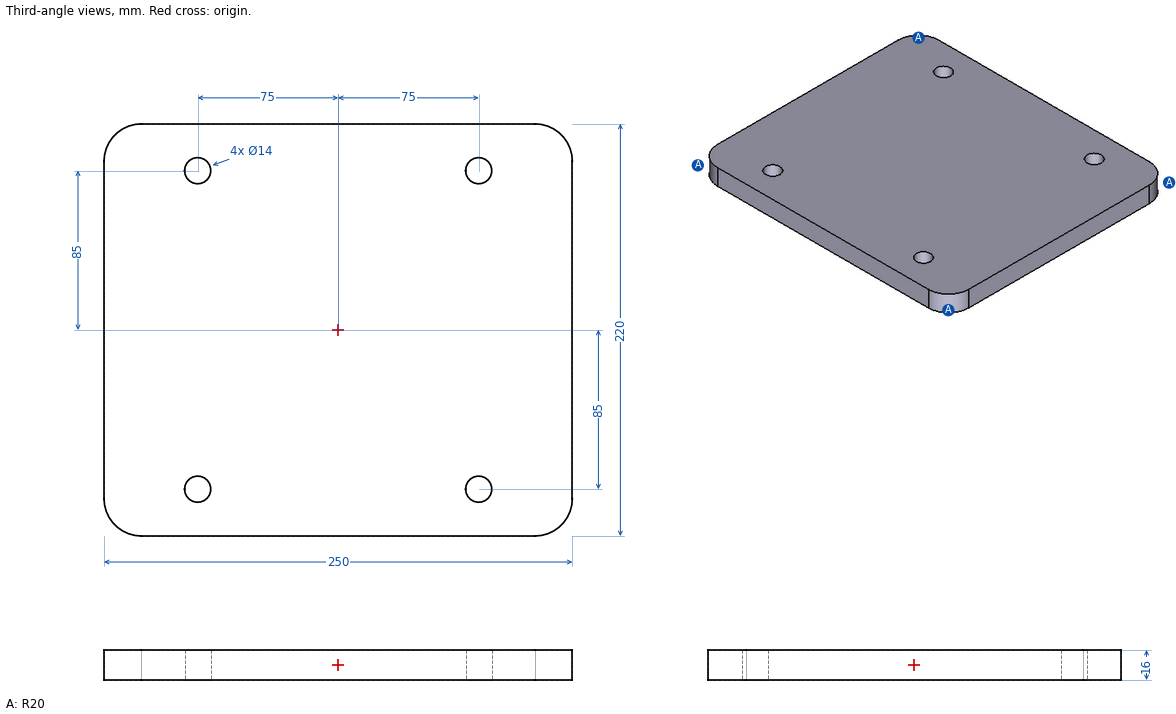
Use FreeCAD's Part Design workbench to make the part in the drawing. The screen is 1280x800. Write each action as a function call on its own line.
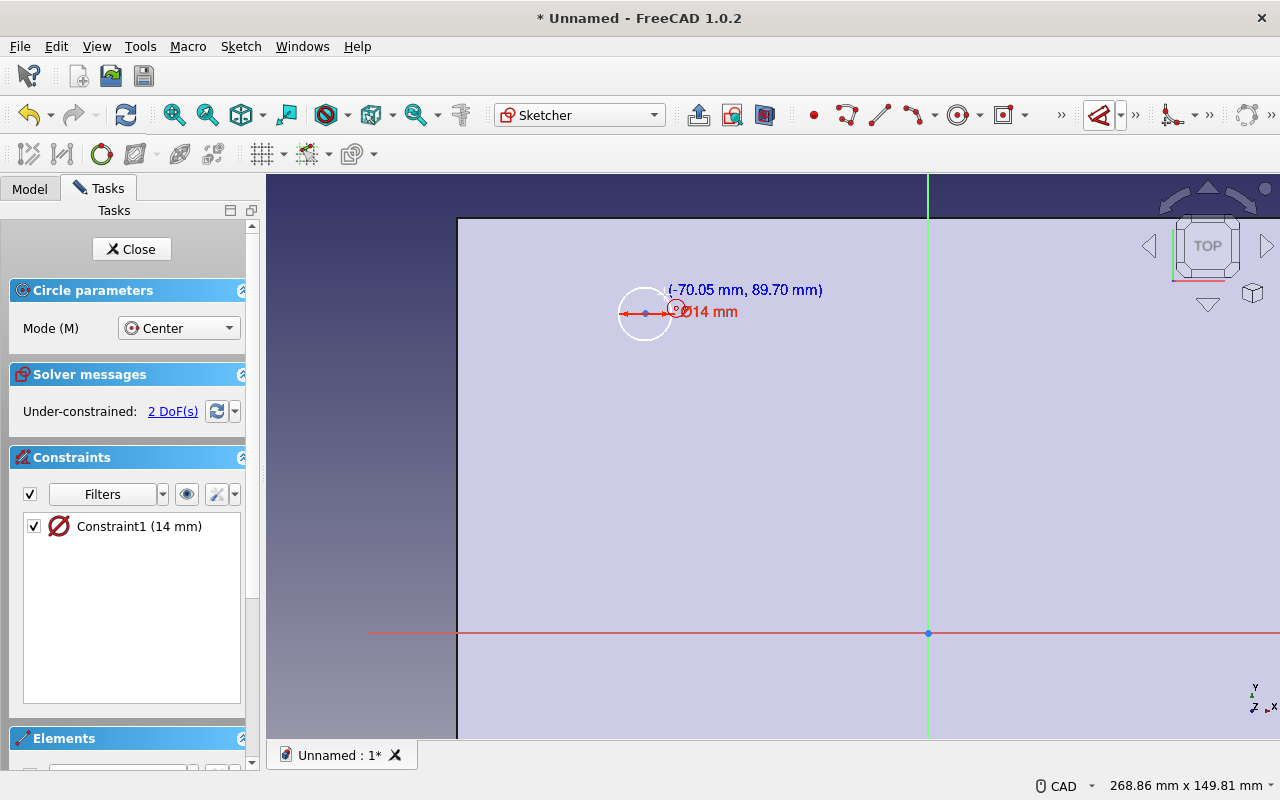
scroll(432, 241, down, 3)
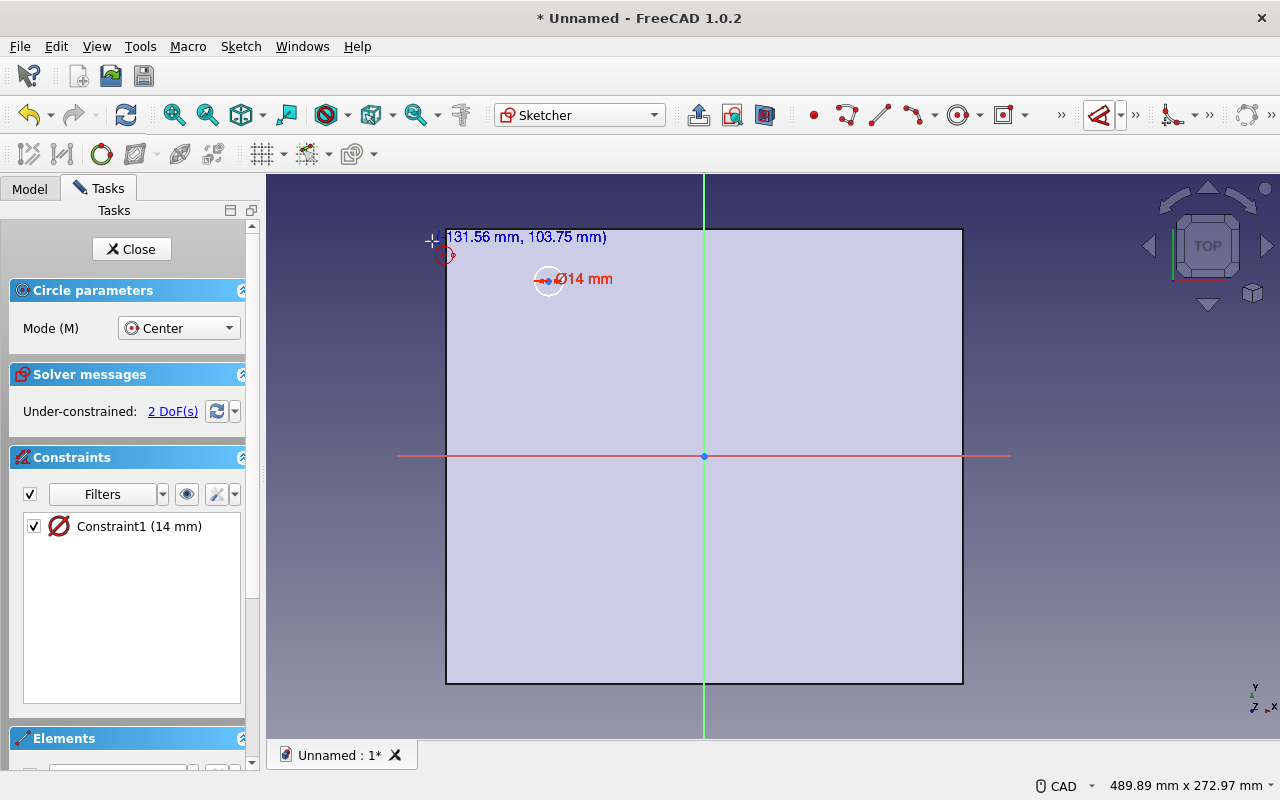
scroll(860, 280, up, 3)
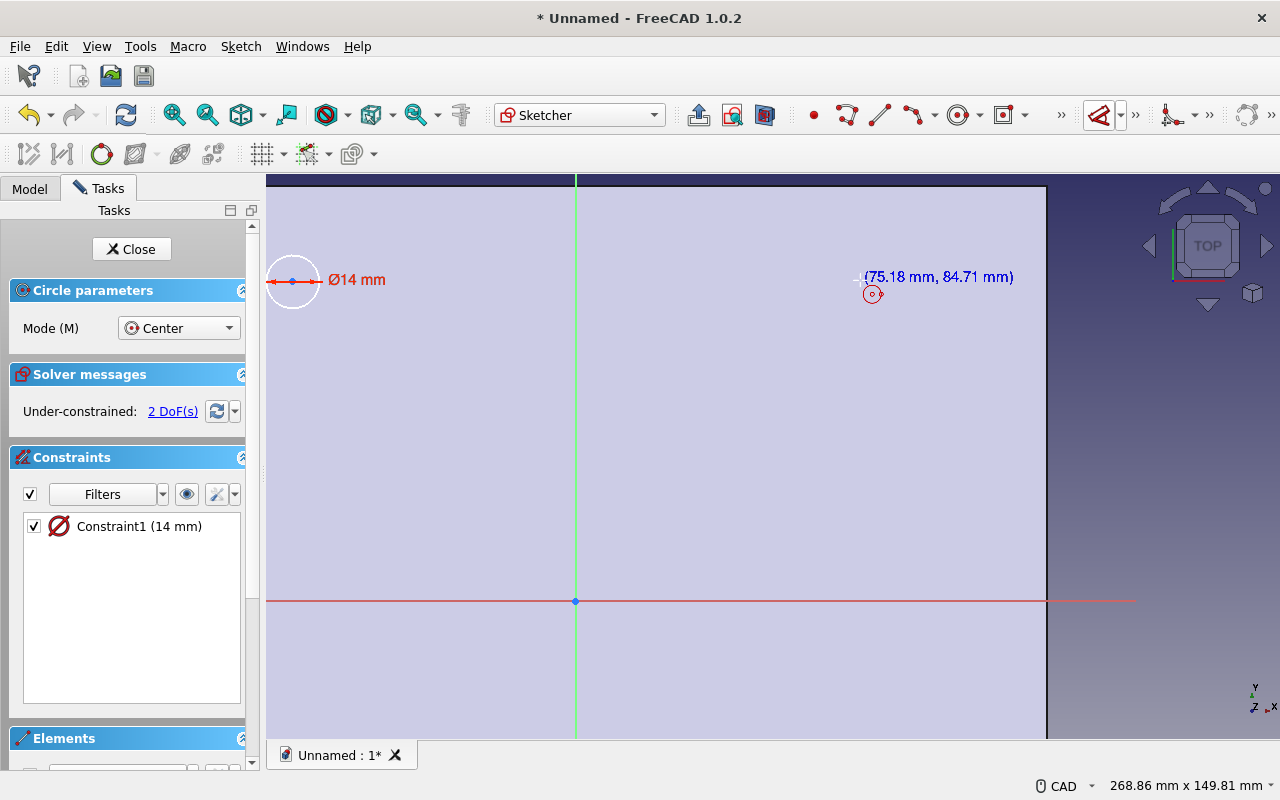
click(859, 281)
move(878, 262)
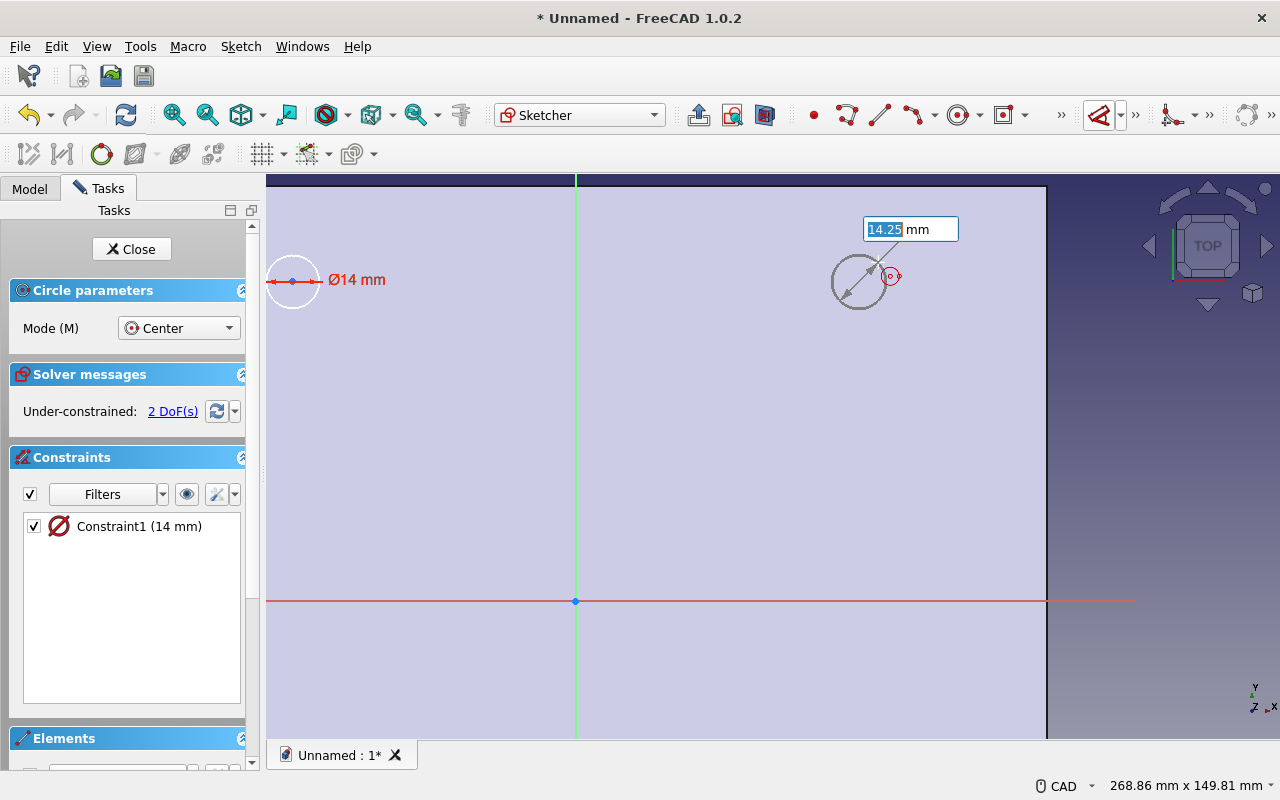
text(14)
key(Return)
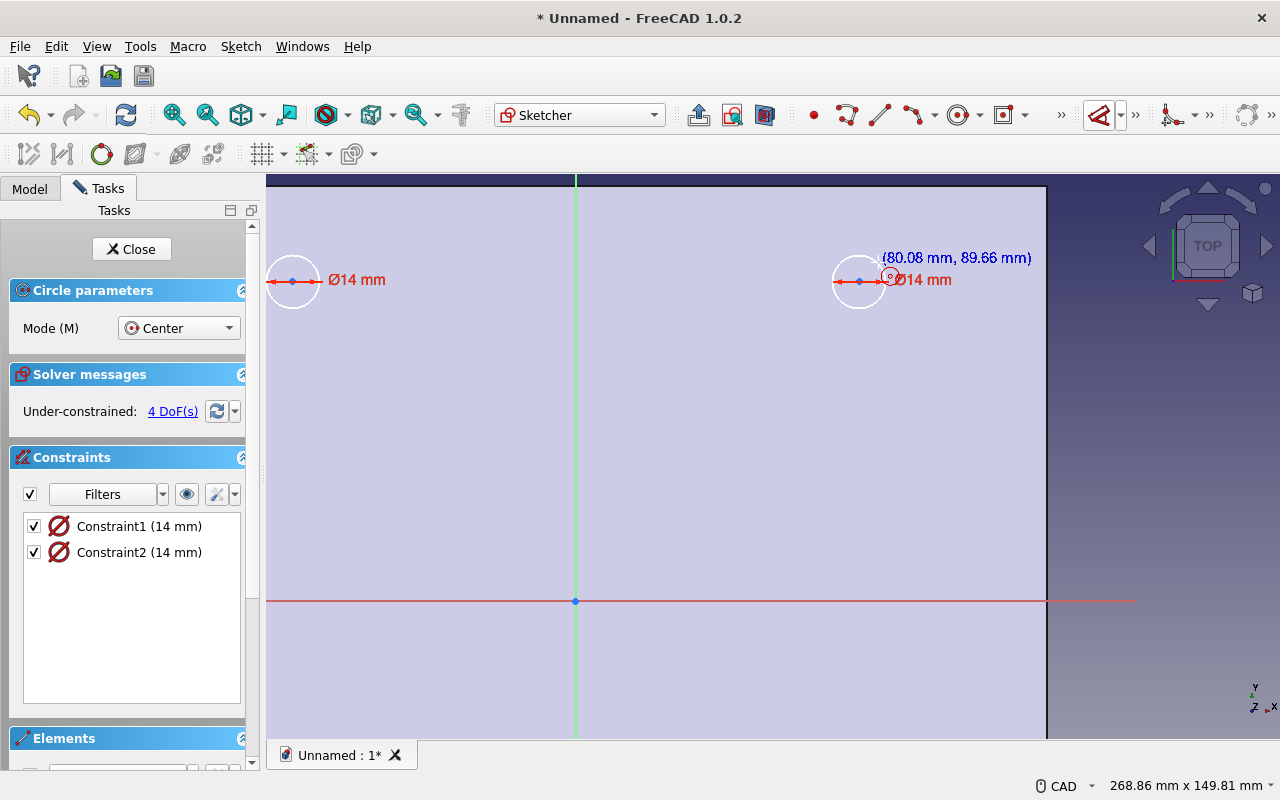
scroll(861, 281, down, 3)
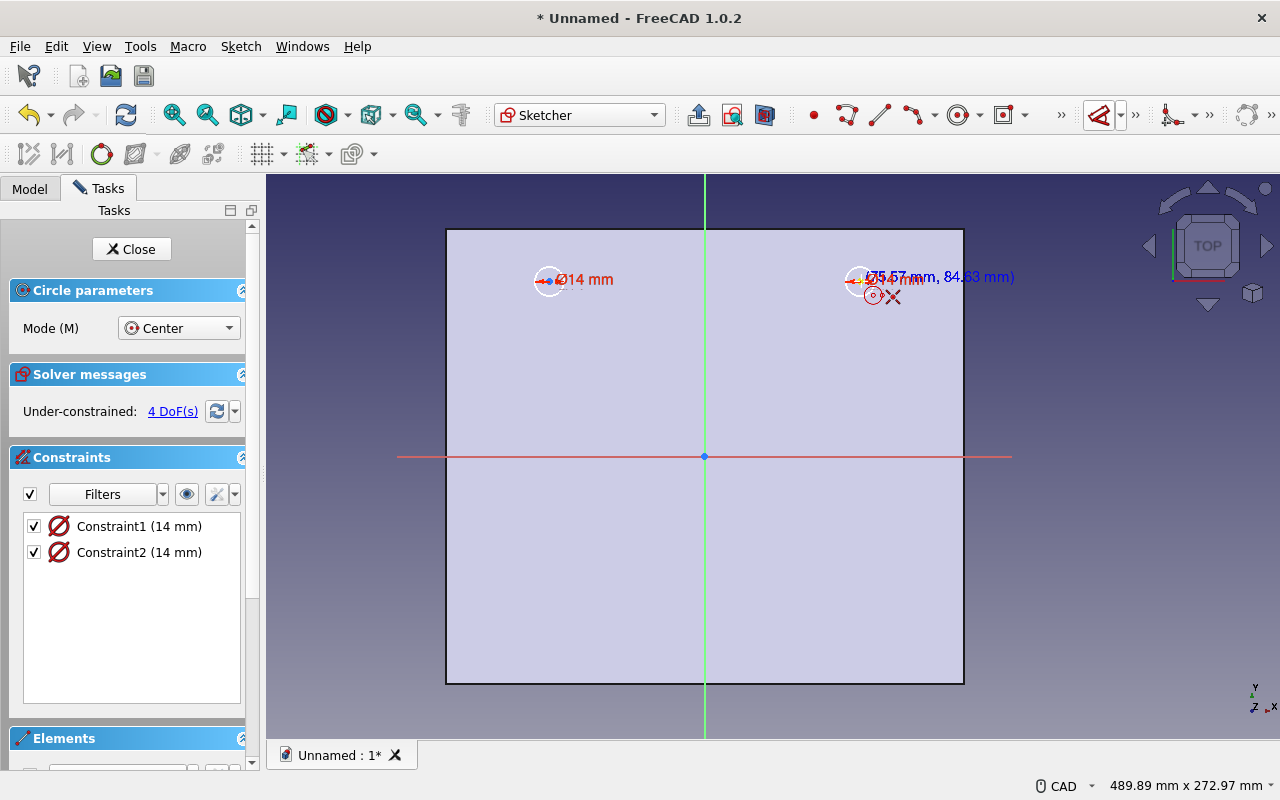
scroll(860, 633, up, 3)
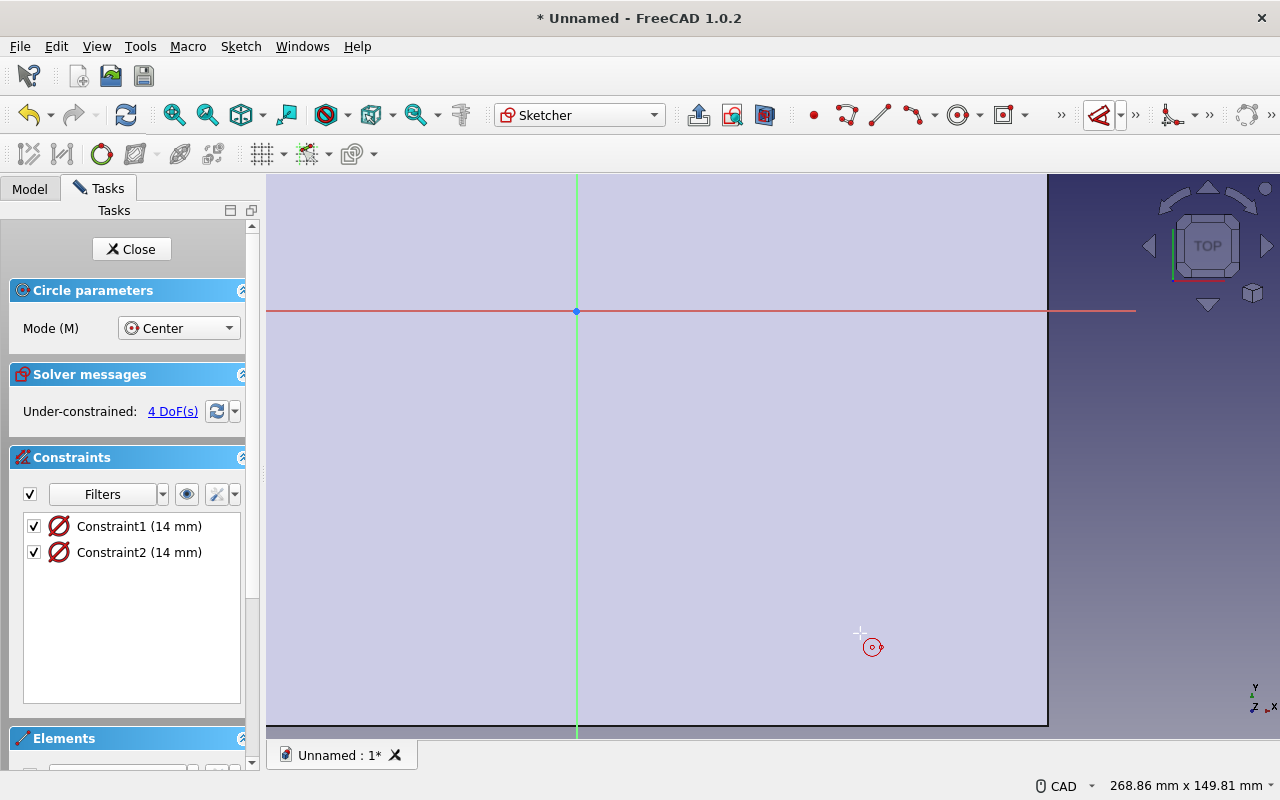
click(860, 632)
move(878, 613)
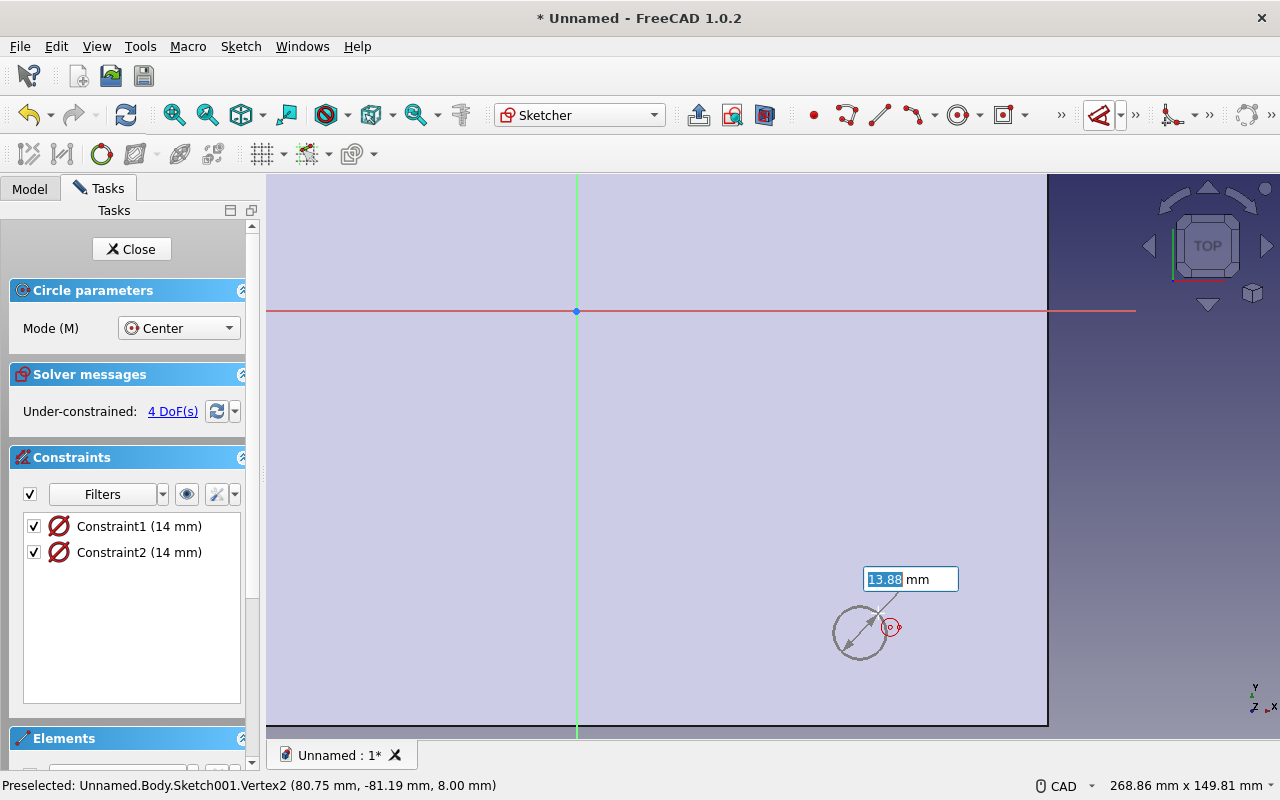
text(14)
key(Return)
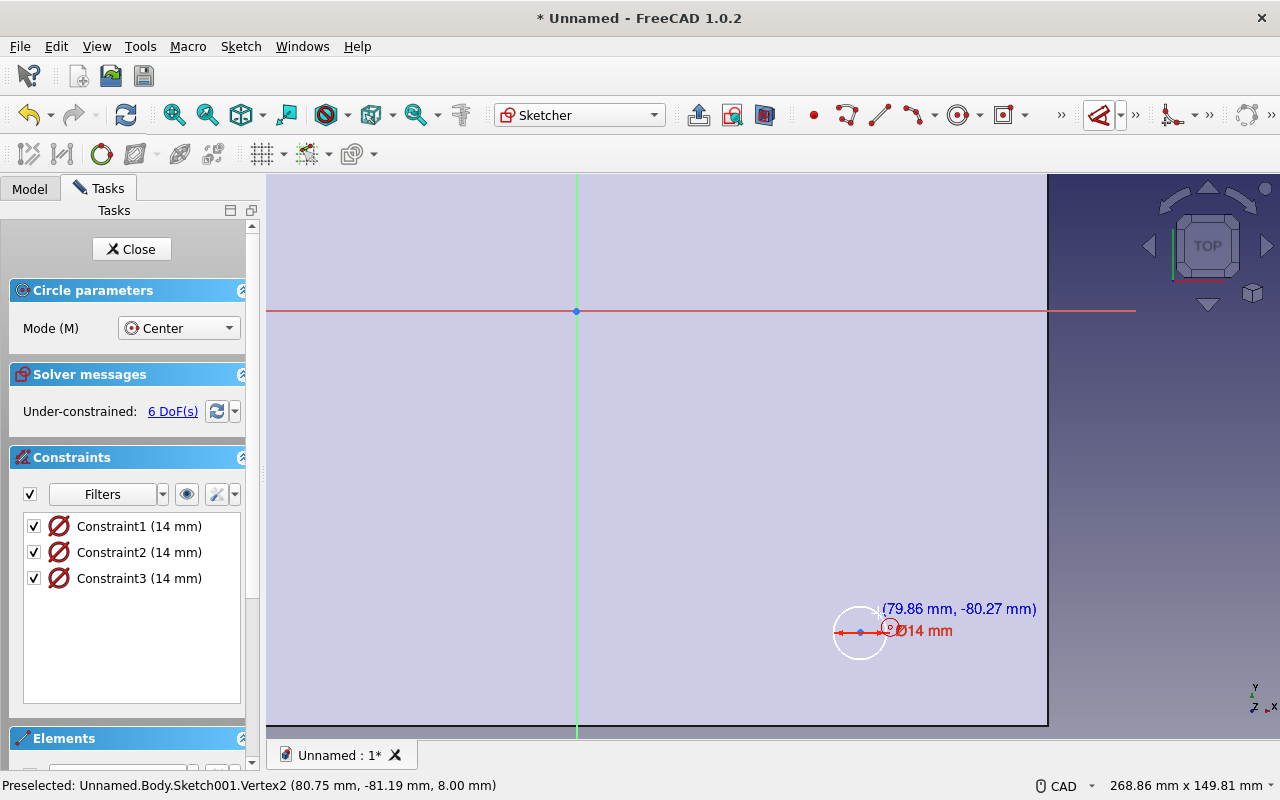
scroll(860, 633, down, 3)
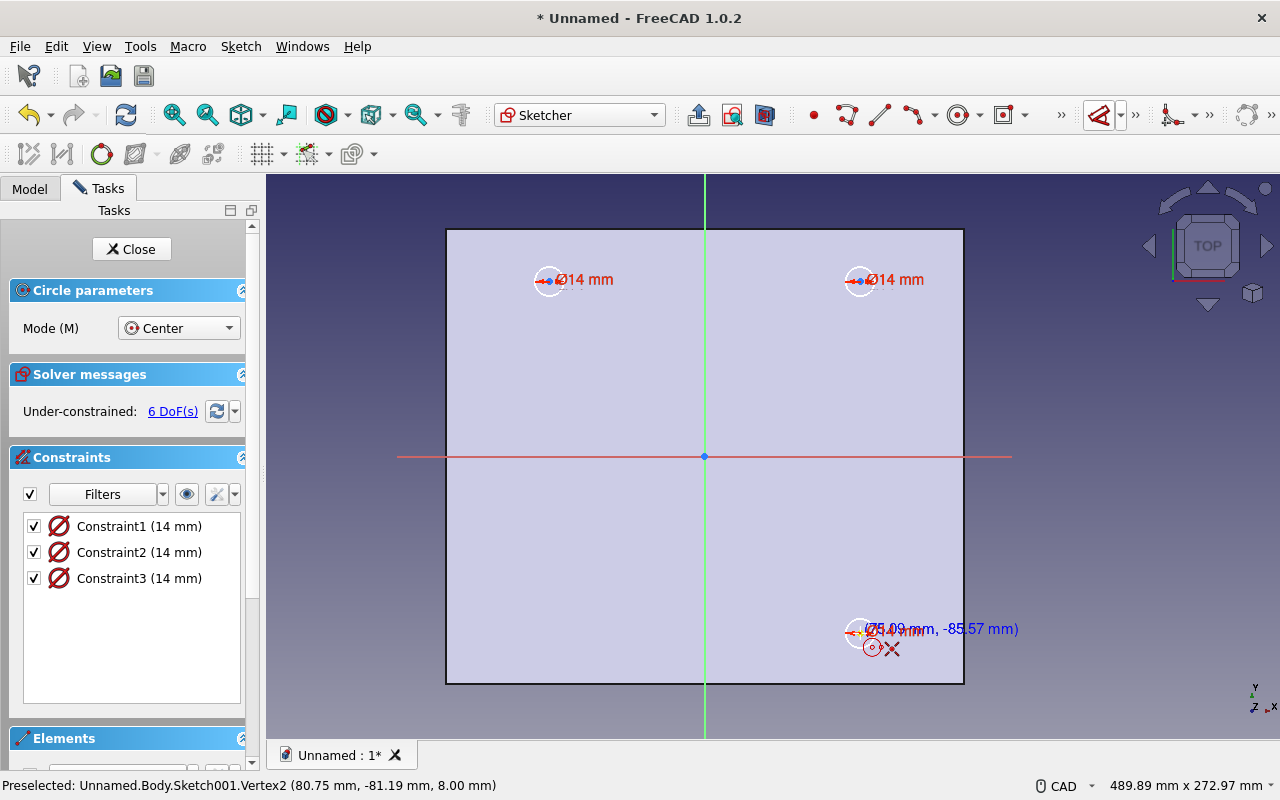
scroll(550, 633, up, 3)